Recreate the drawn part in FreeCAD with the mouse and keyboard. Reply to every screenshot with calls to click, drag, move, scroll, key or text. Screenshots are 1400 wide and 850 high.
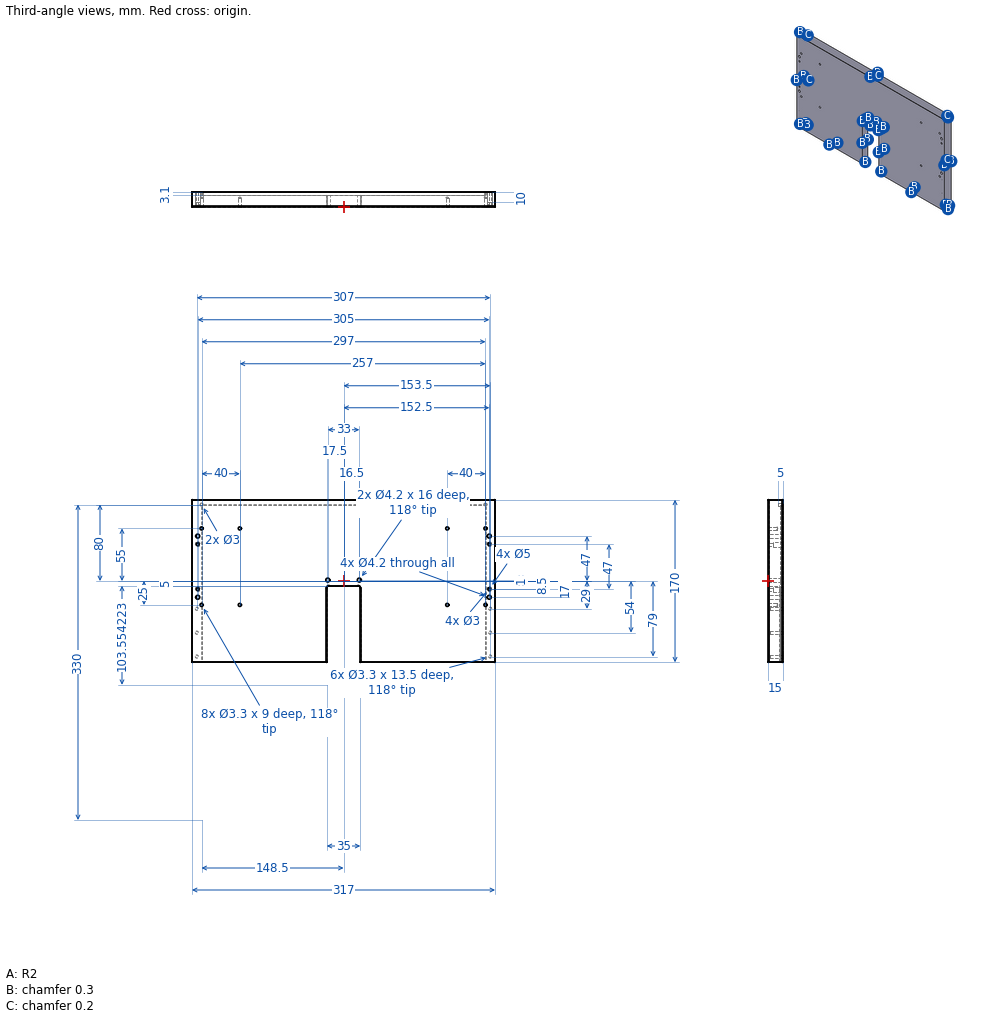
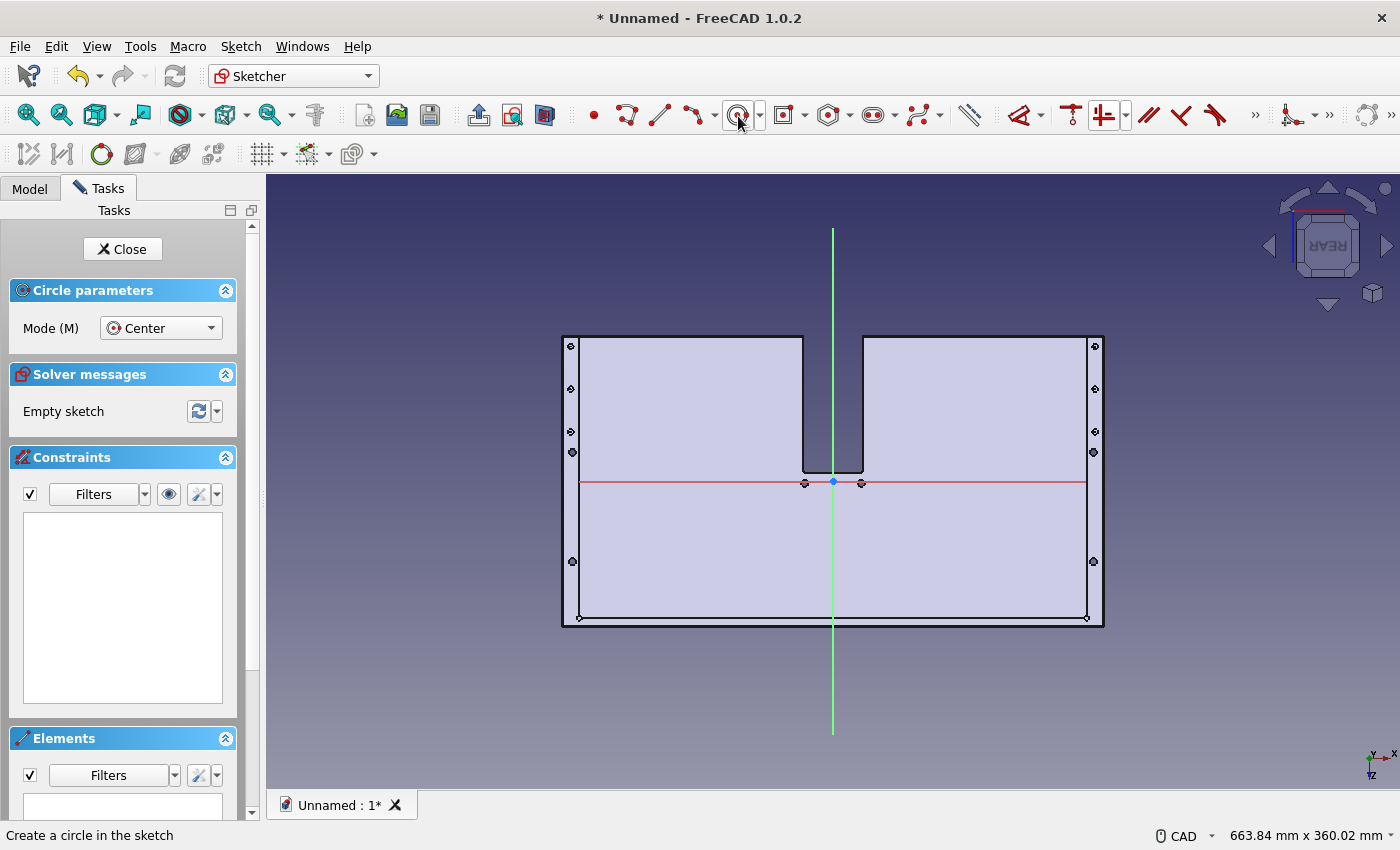
scroll(1094, 467, up, 9)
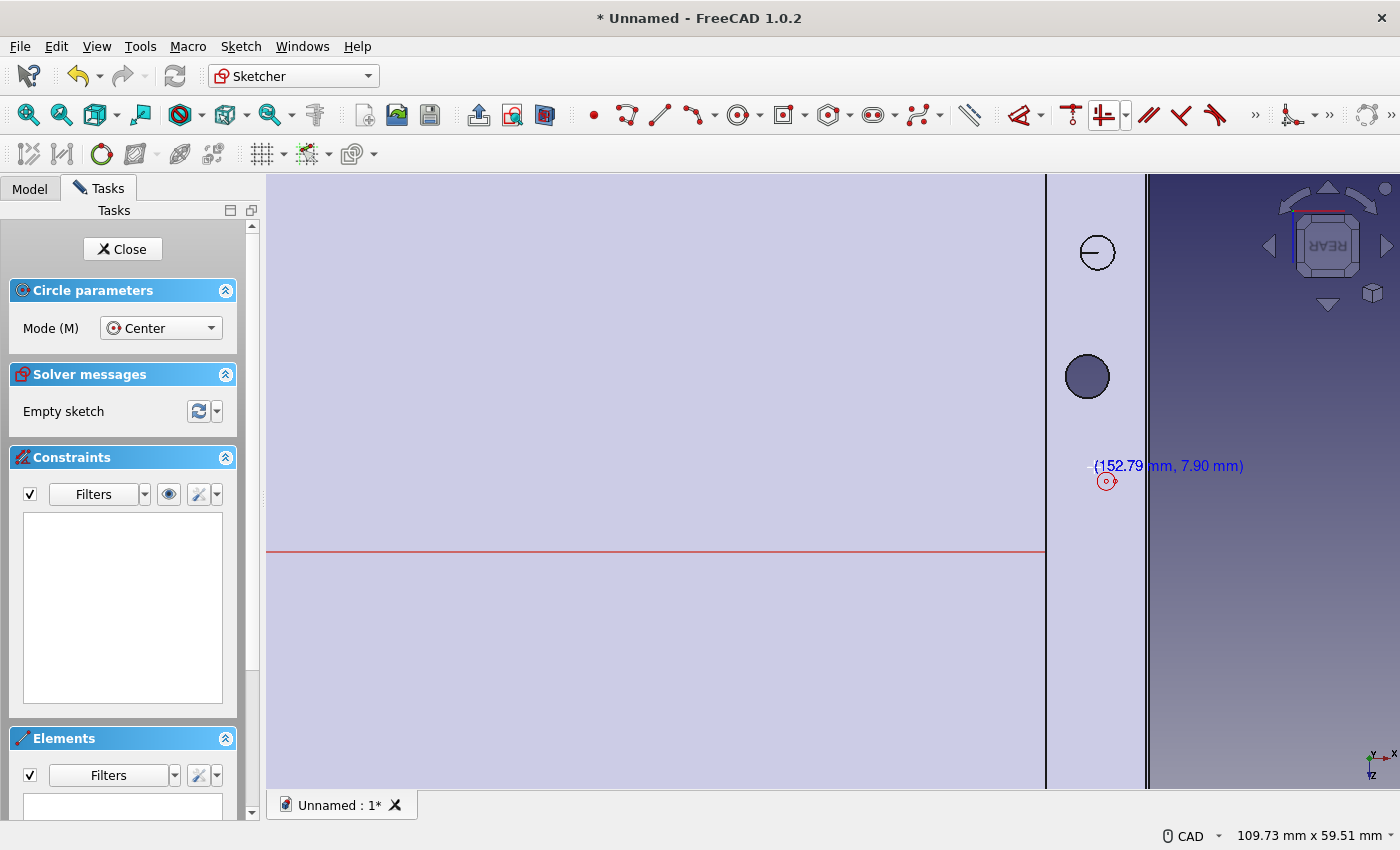
scroll(1082, 424, down, 8)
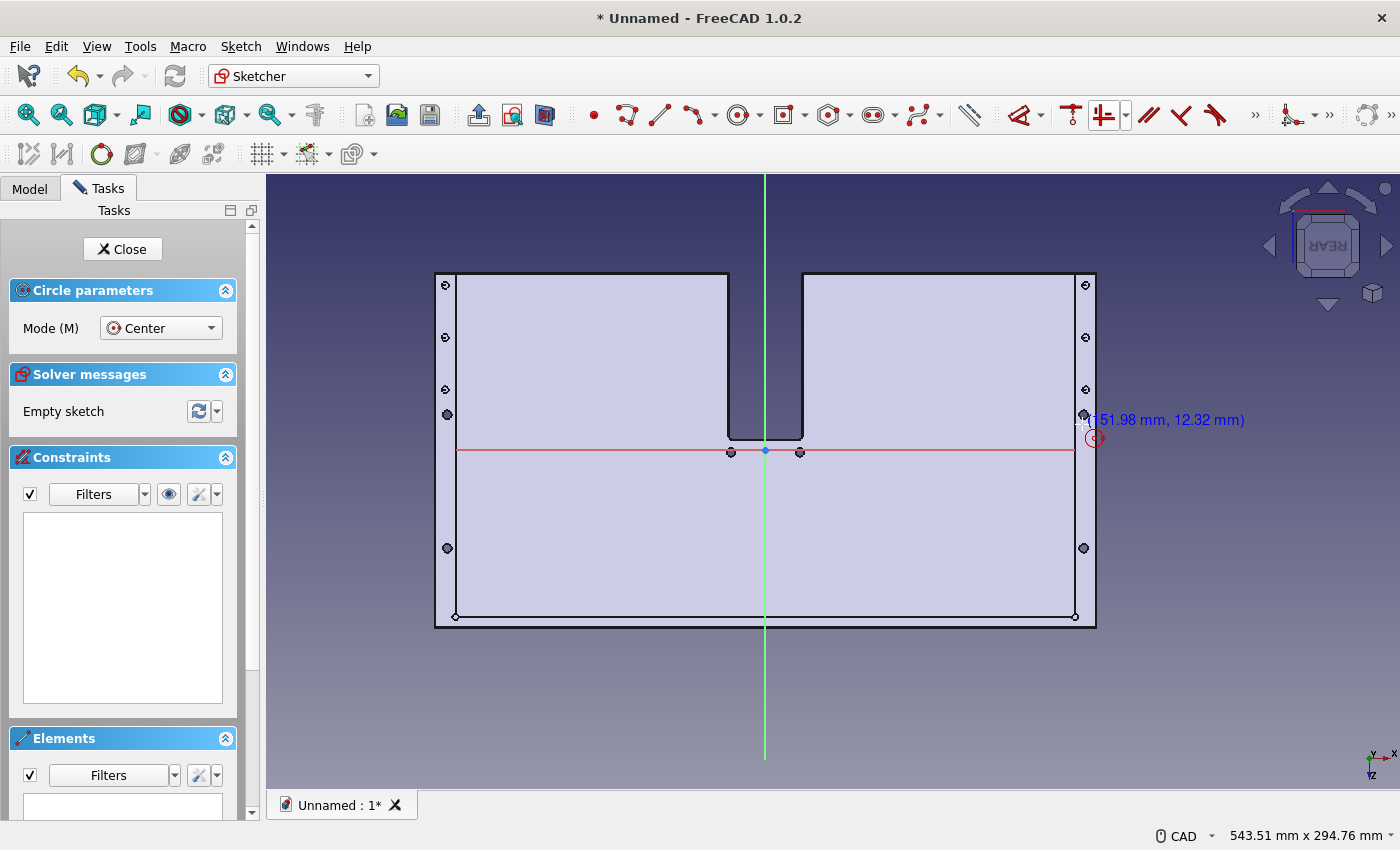
click(1084, 432)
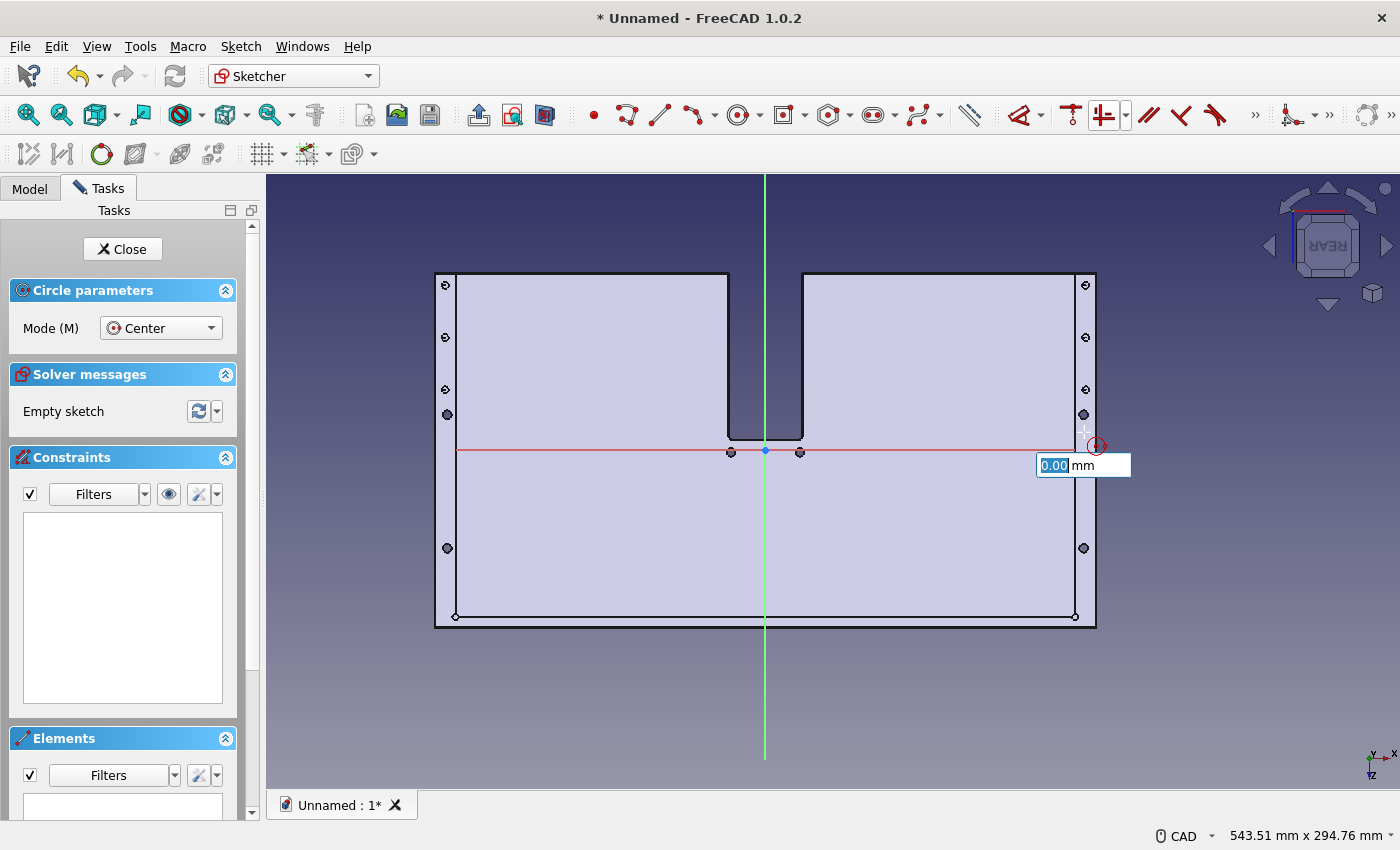
scroll(1087, 429, up, 6)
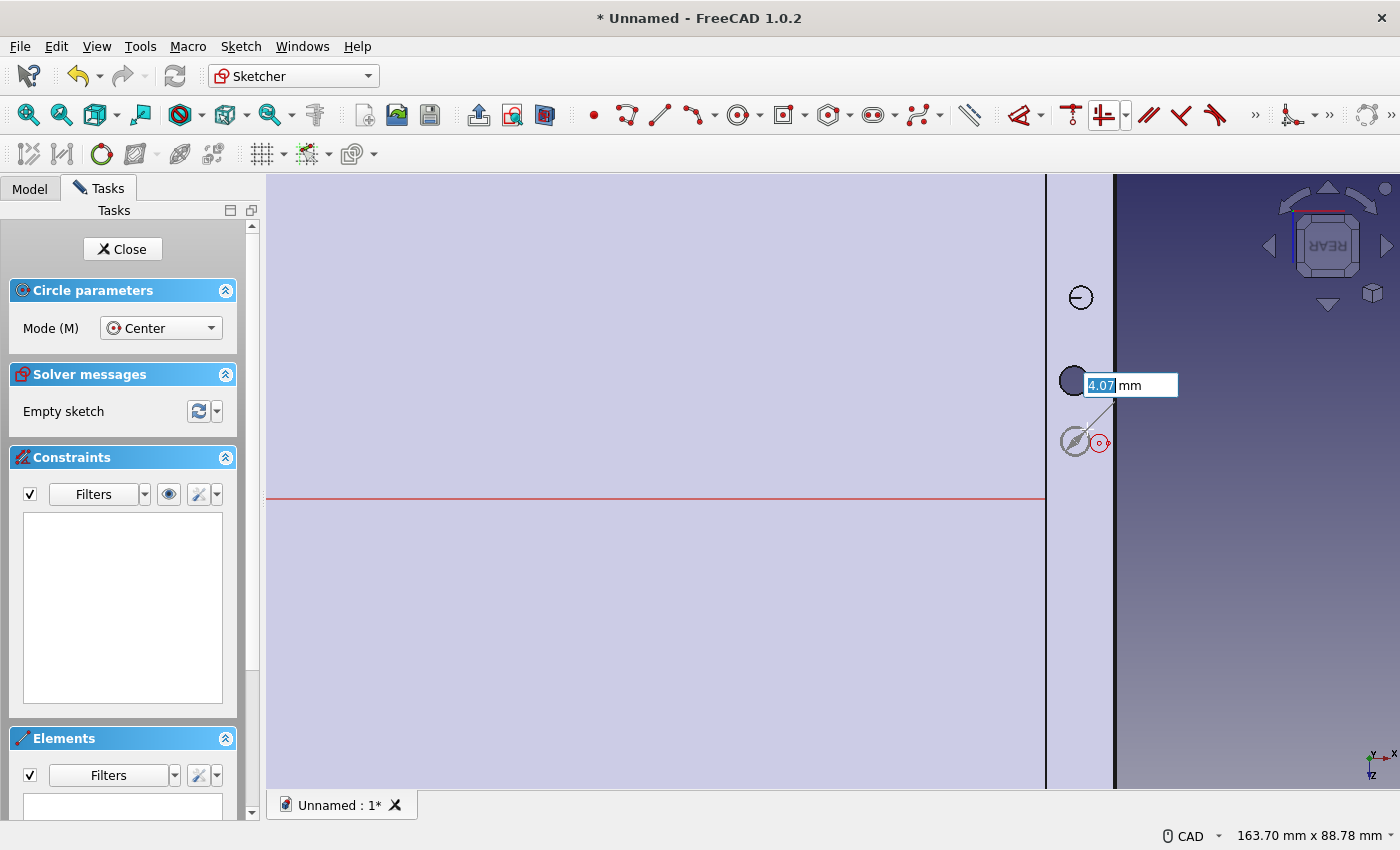
click(1086, 427)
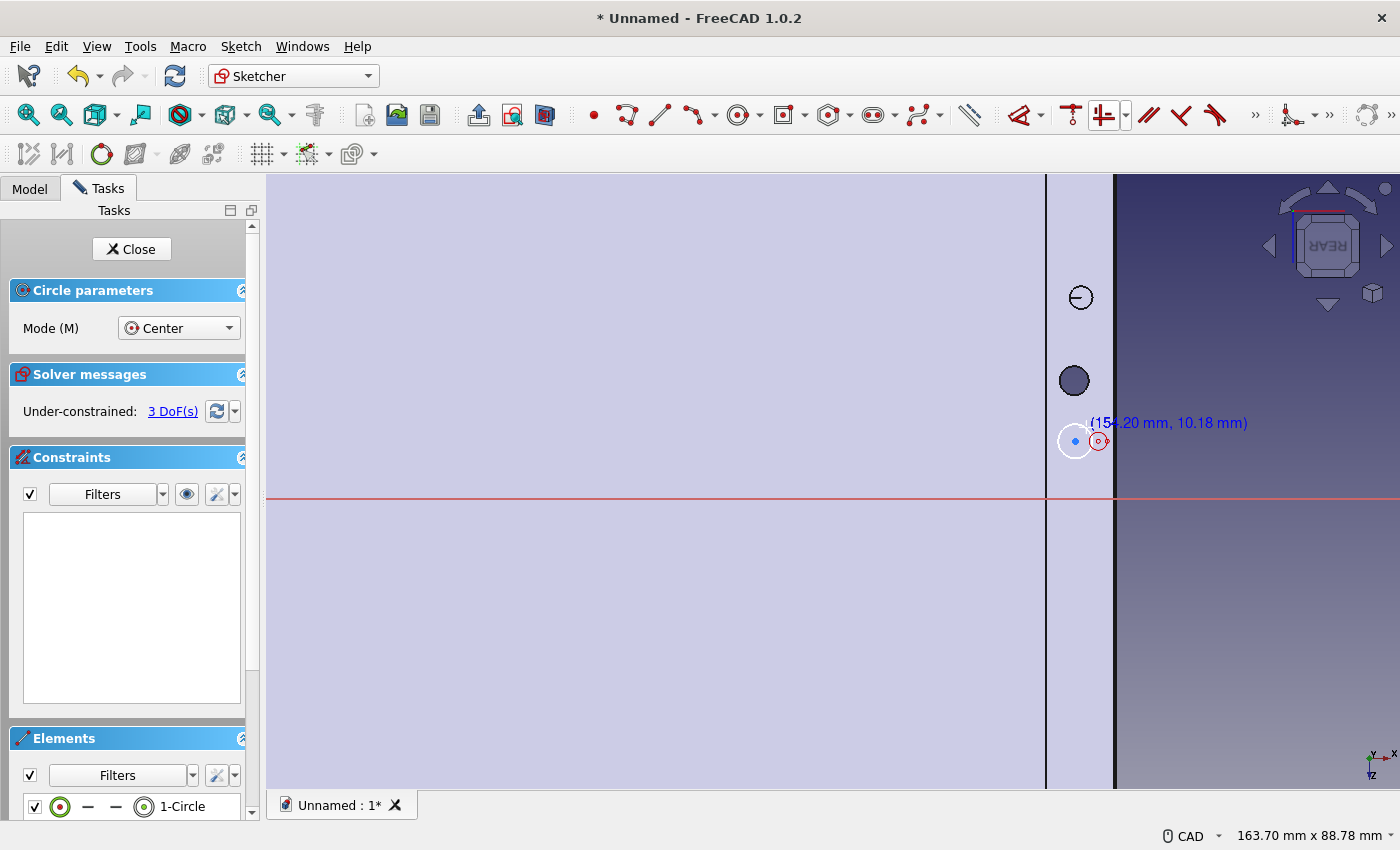
scroll(1086, 429, down, 6)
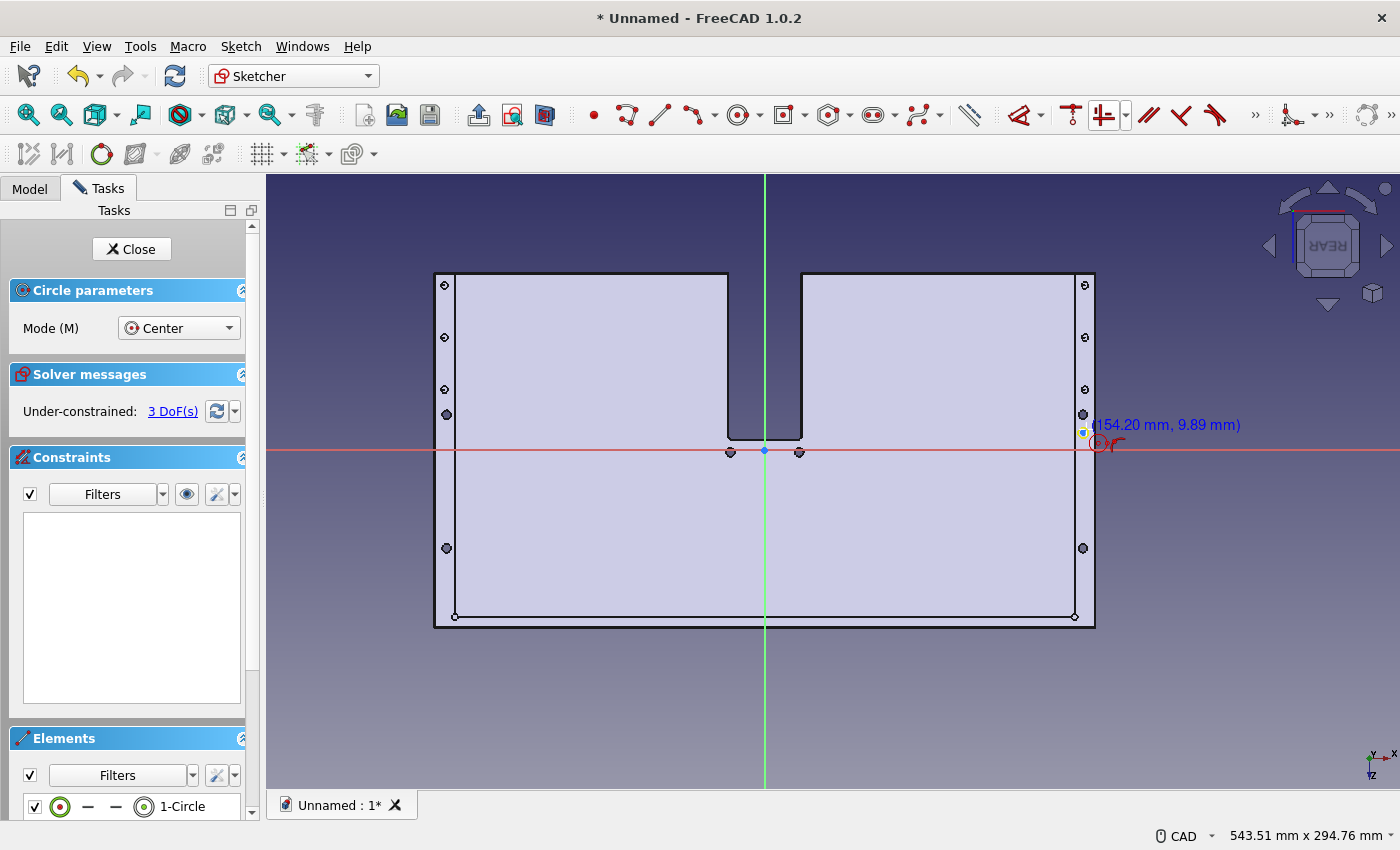
scroll(1083, 531, up, 8)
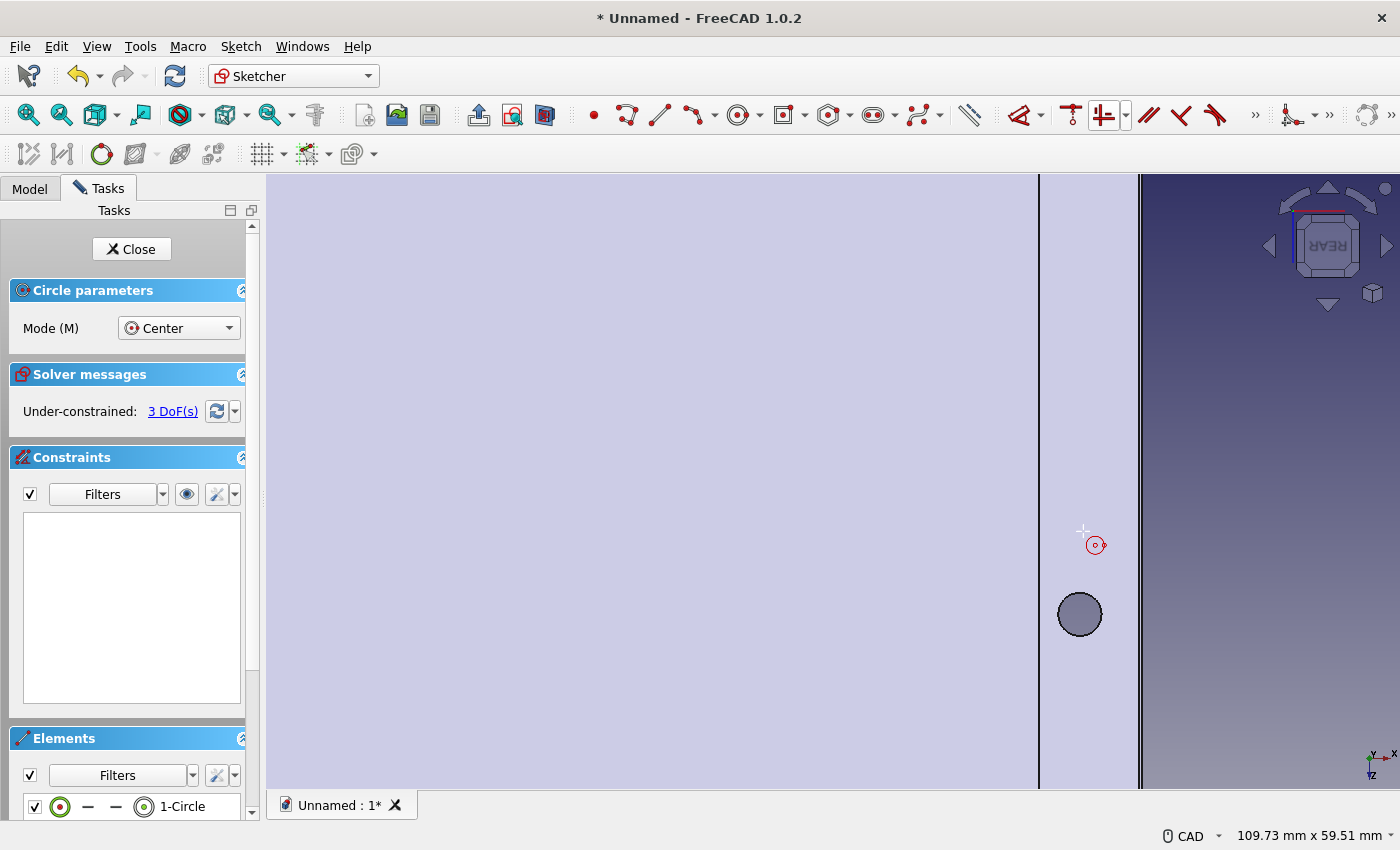
scroll(1083, 532, down, 8)